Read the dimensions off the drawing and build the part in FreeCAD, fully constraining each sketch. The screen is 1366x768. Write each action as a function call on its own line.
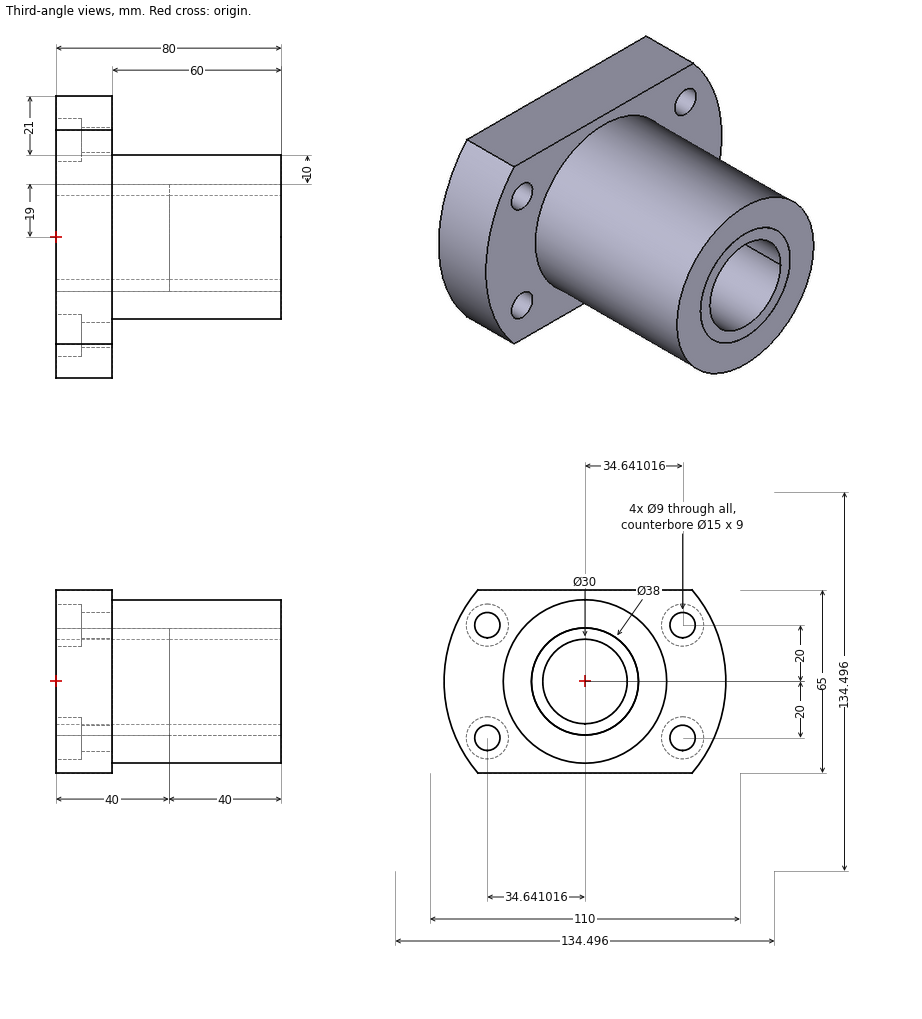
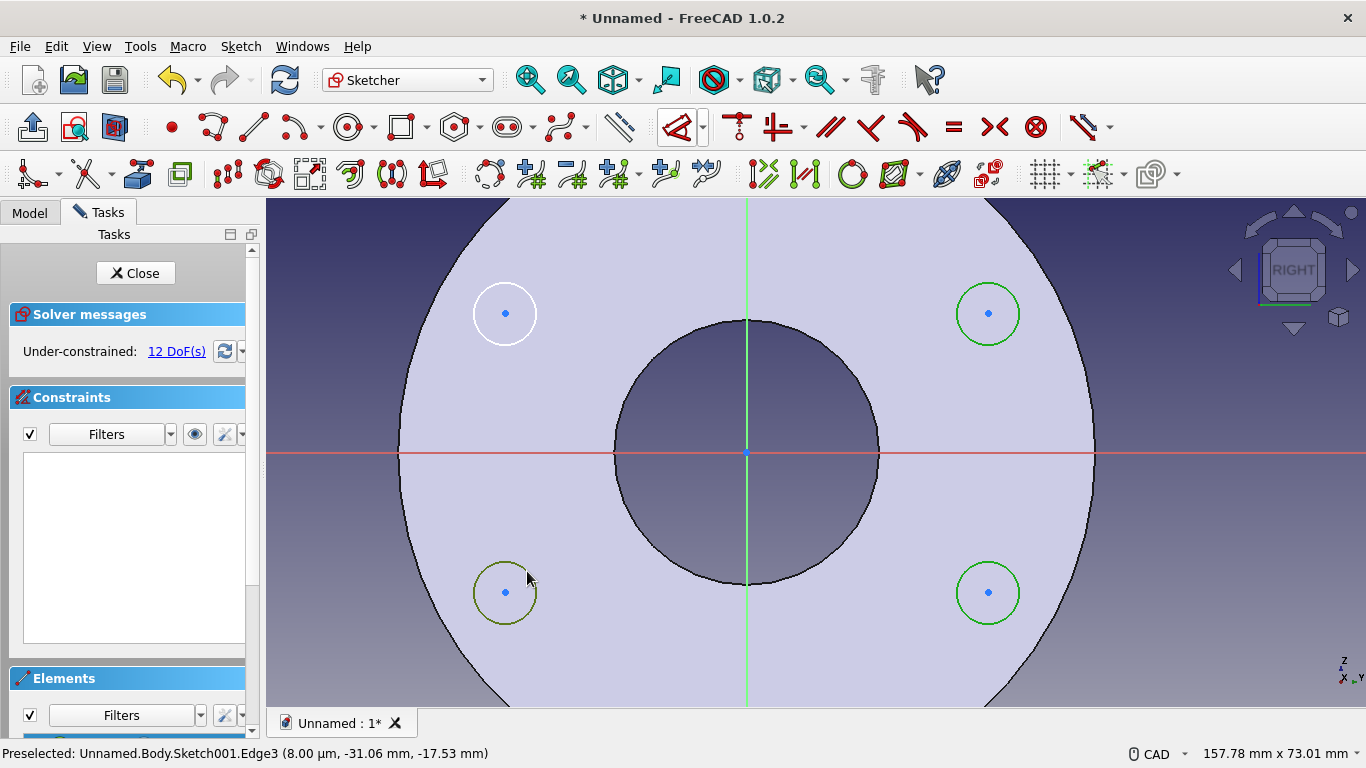
click(527, 292)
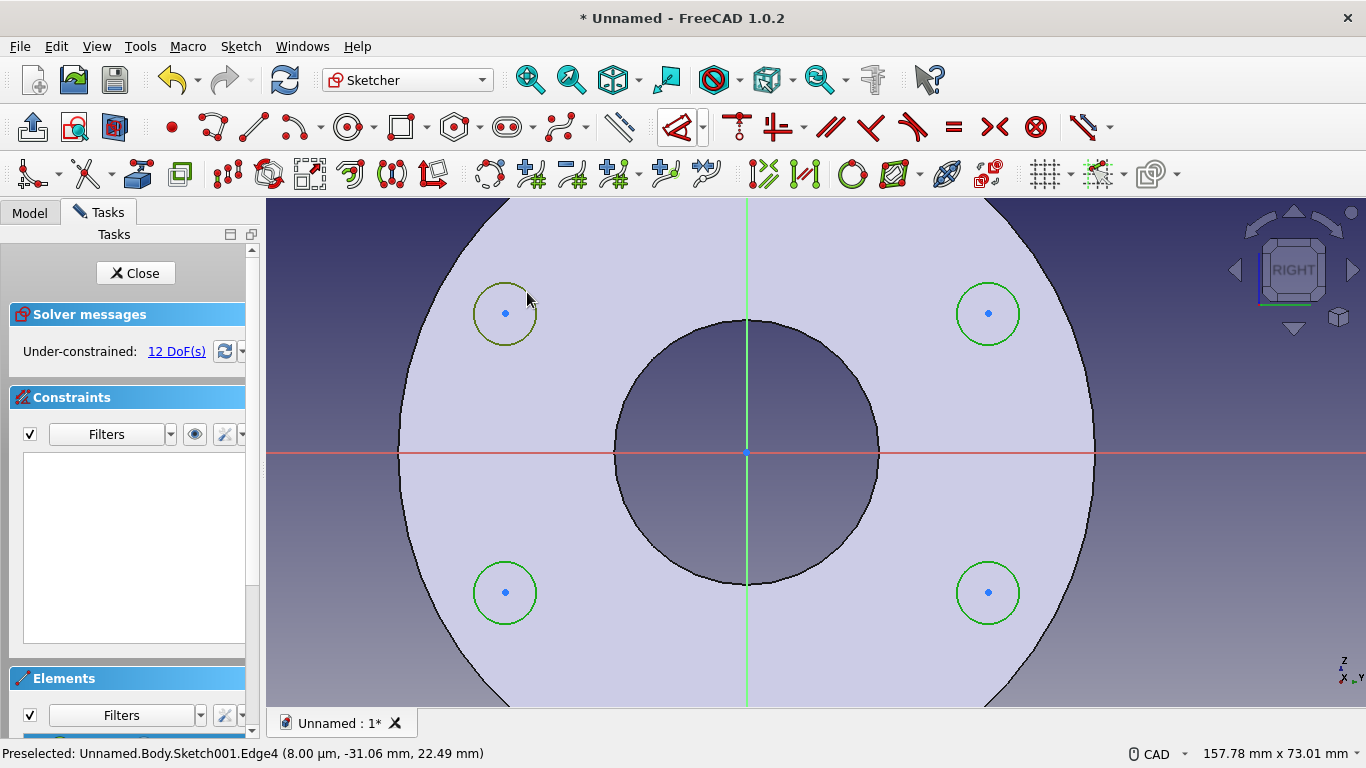
click(954, 128)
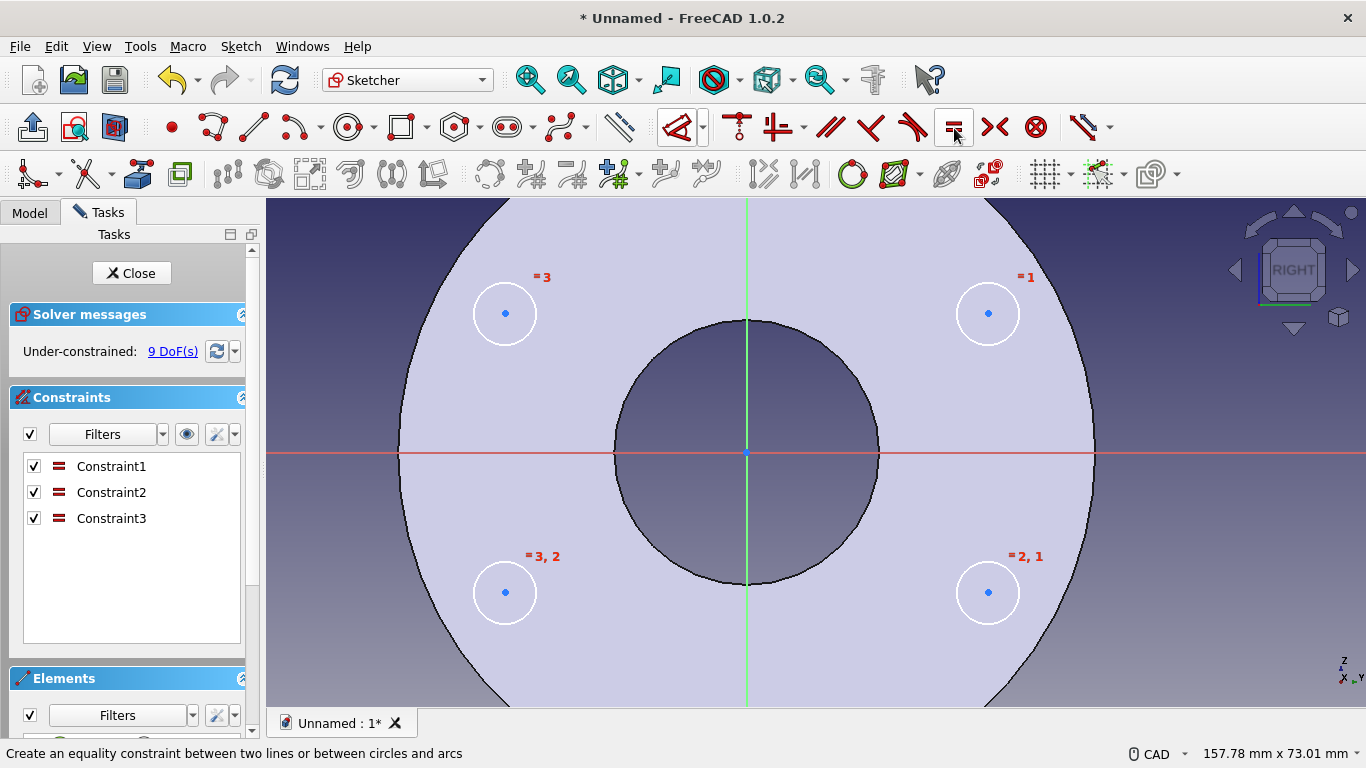
click(988, 314)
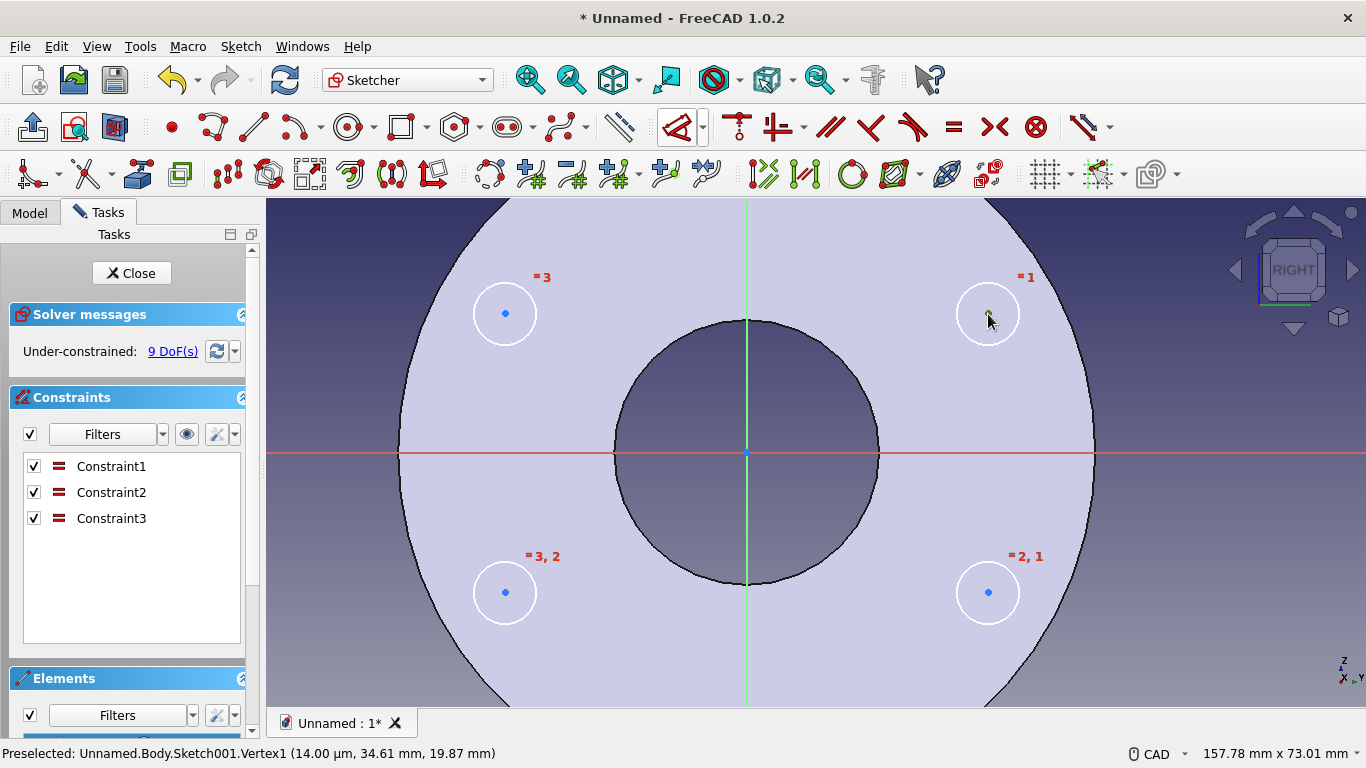
click(988, 593)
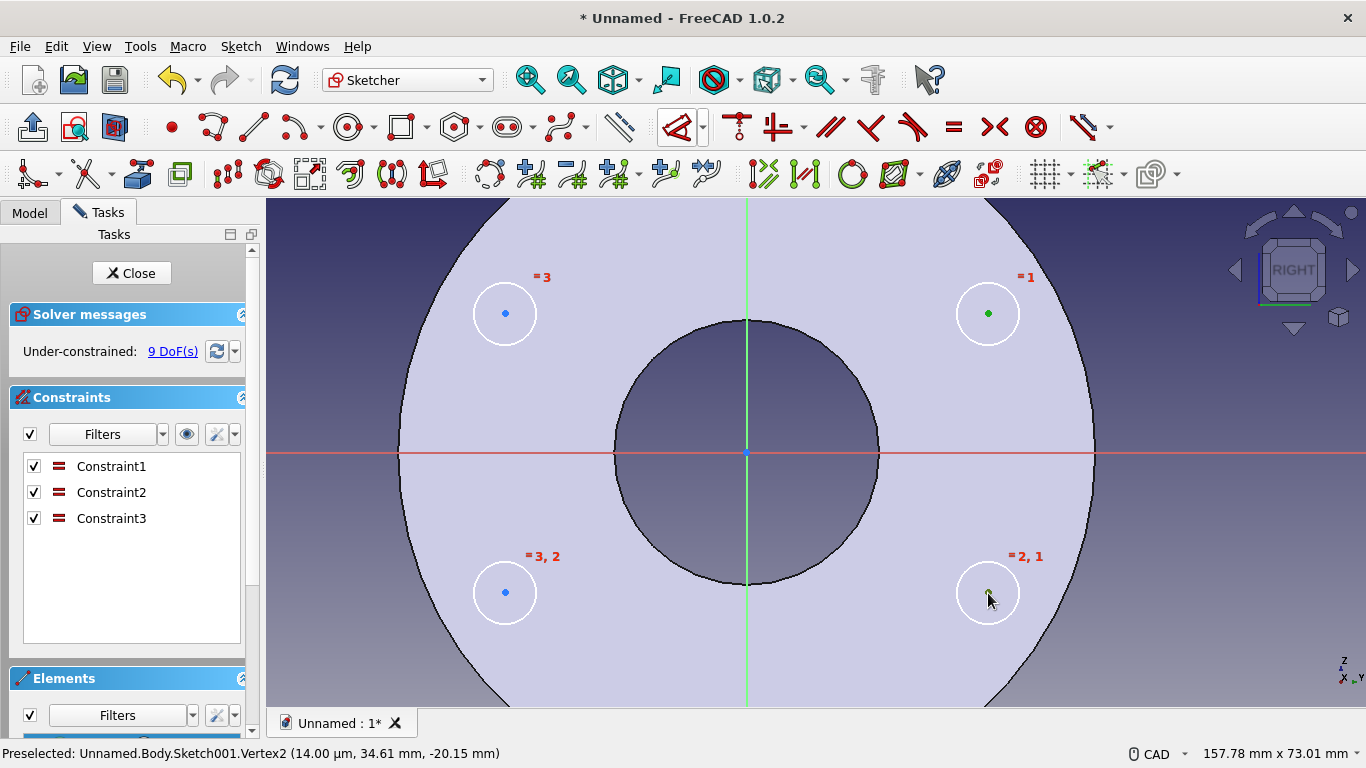
key(v)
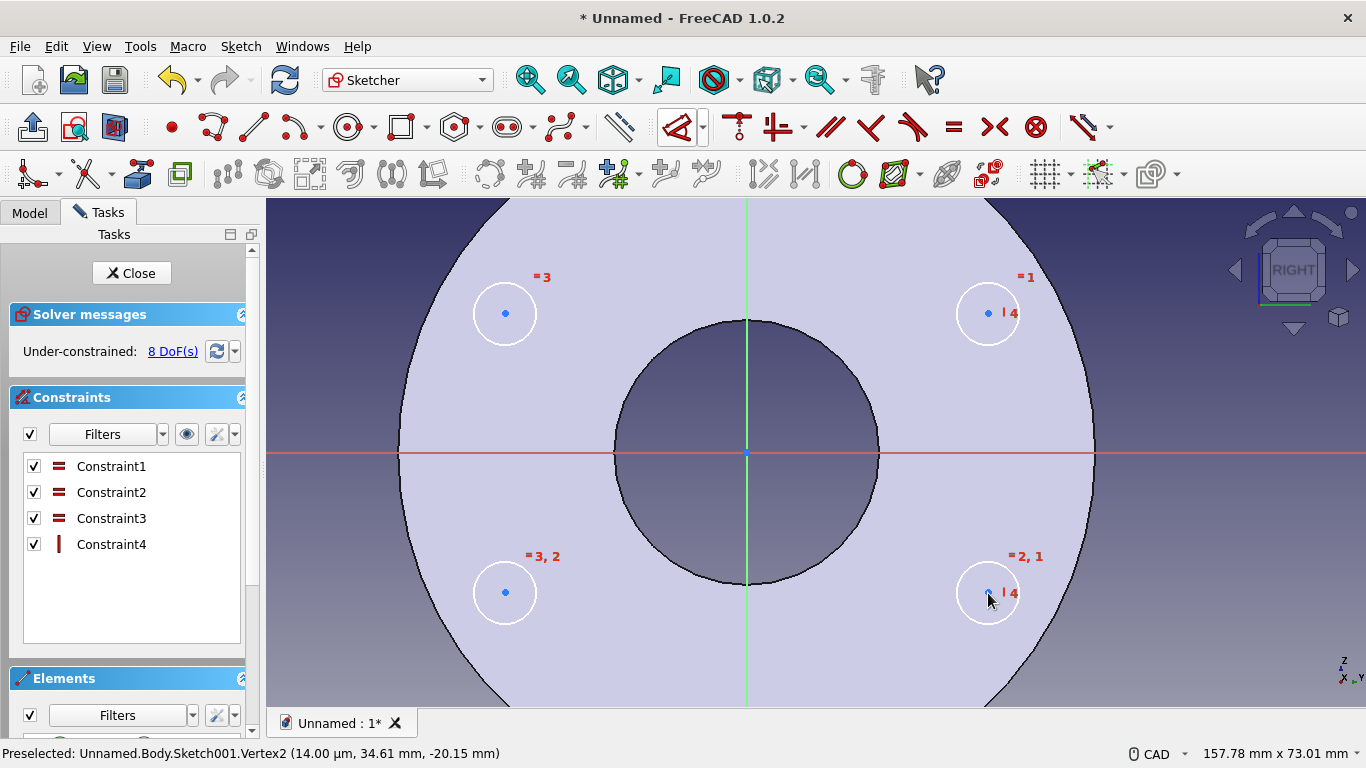
click(988, 593)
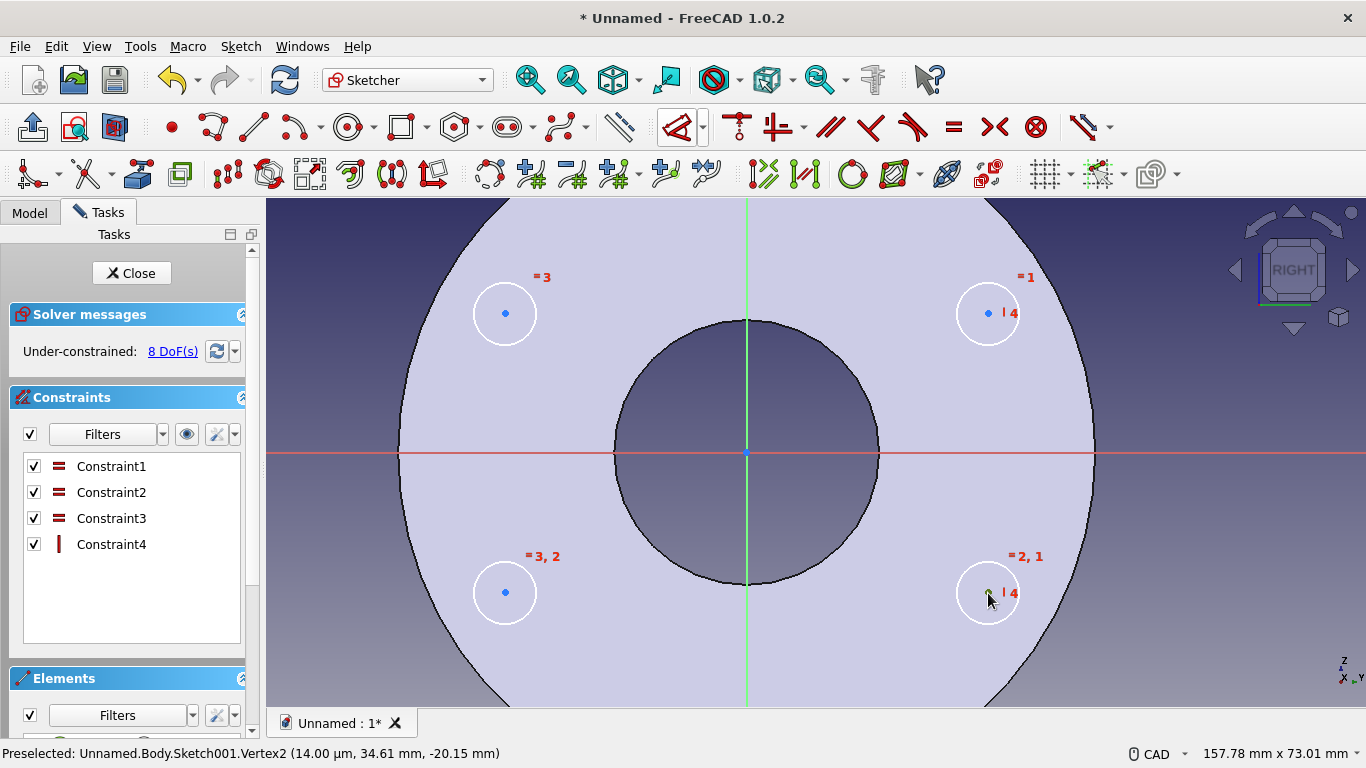
click(505, 593)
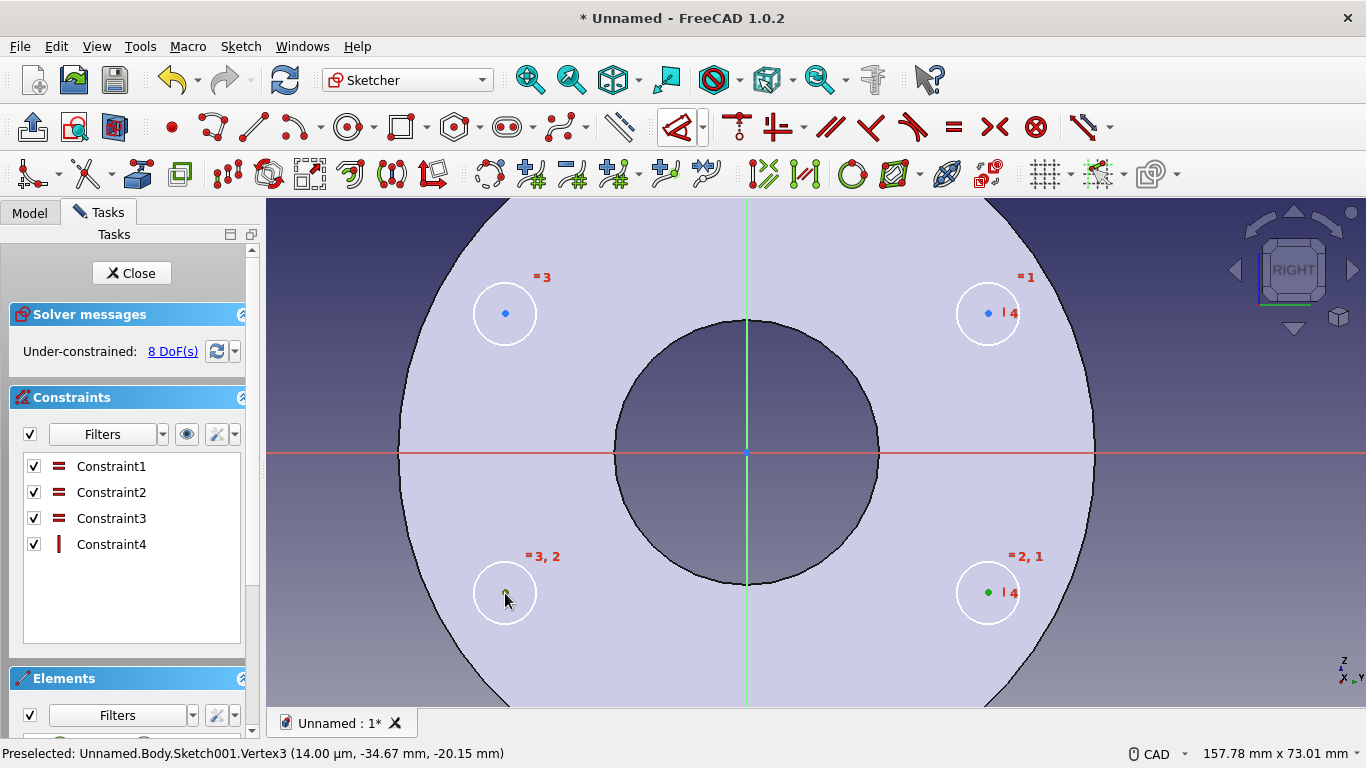
key(h)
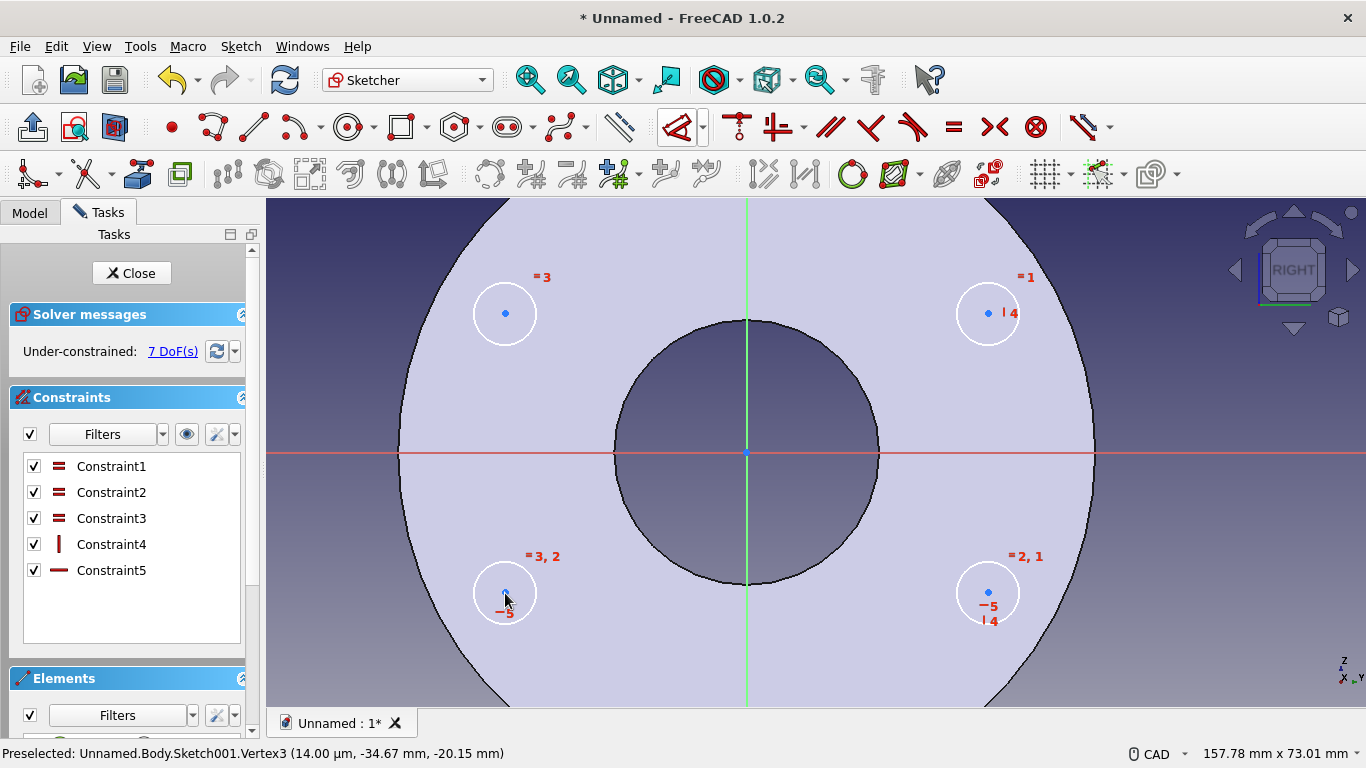
click(505, 593)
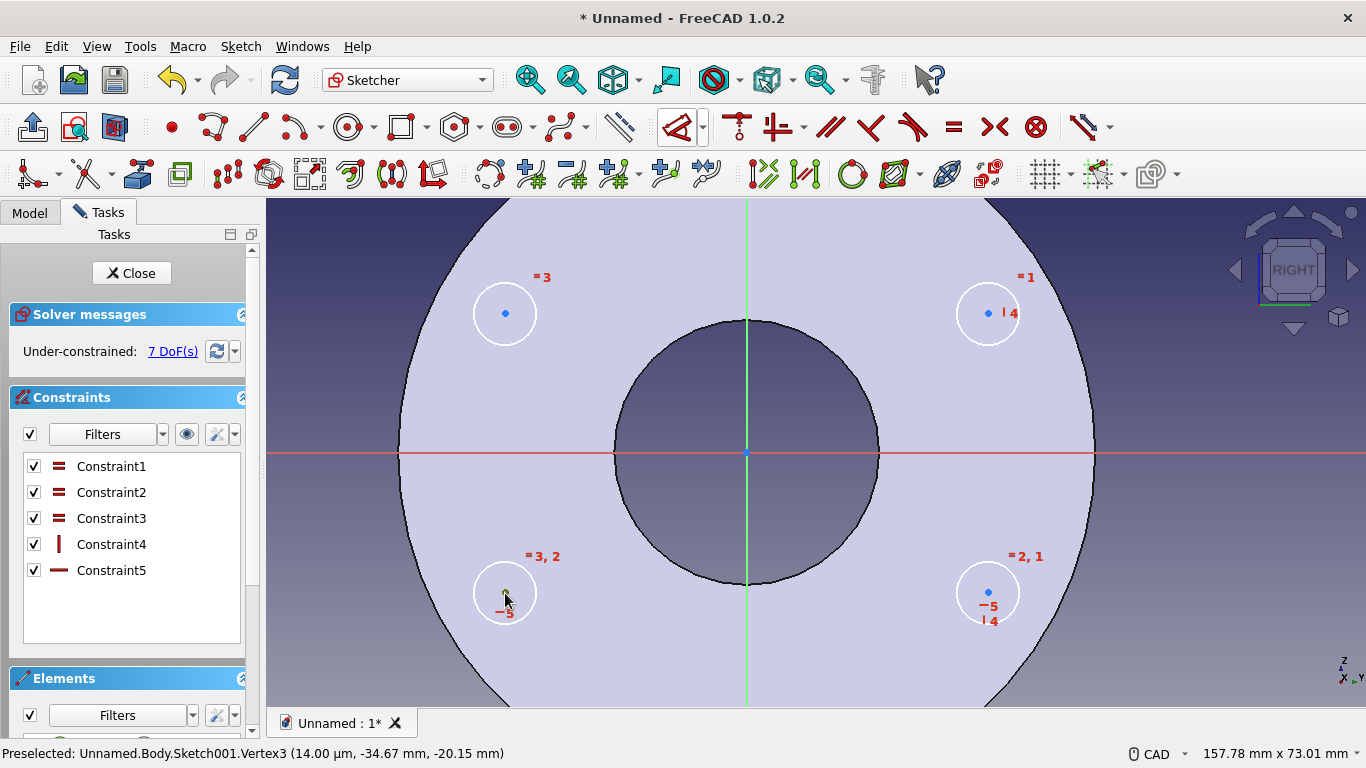
click(505, 314)